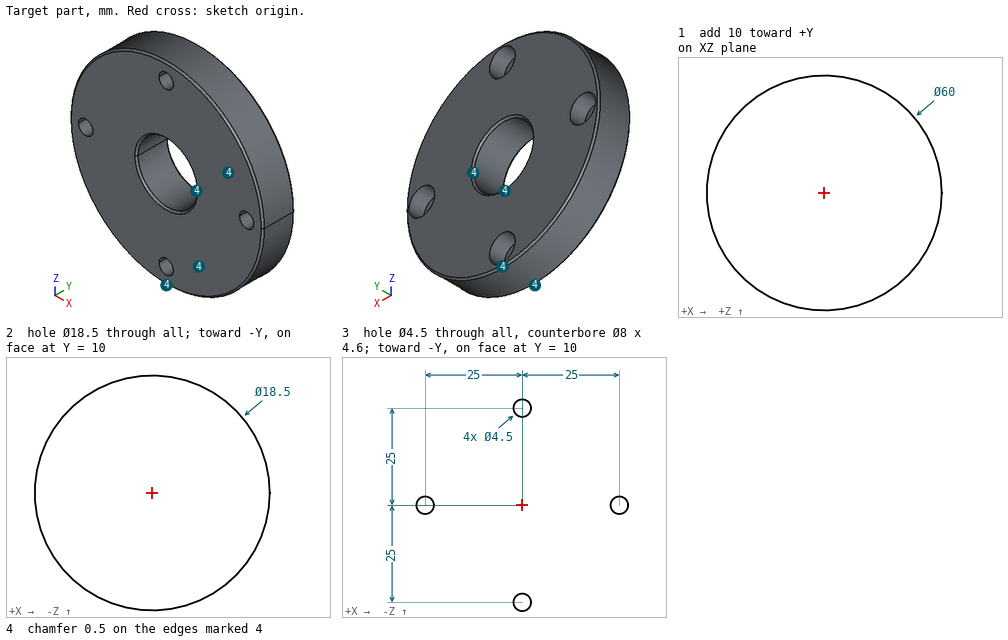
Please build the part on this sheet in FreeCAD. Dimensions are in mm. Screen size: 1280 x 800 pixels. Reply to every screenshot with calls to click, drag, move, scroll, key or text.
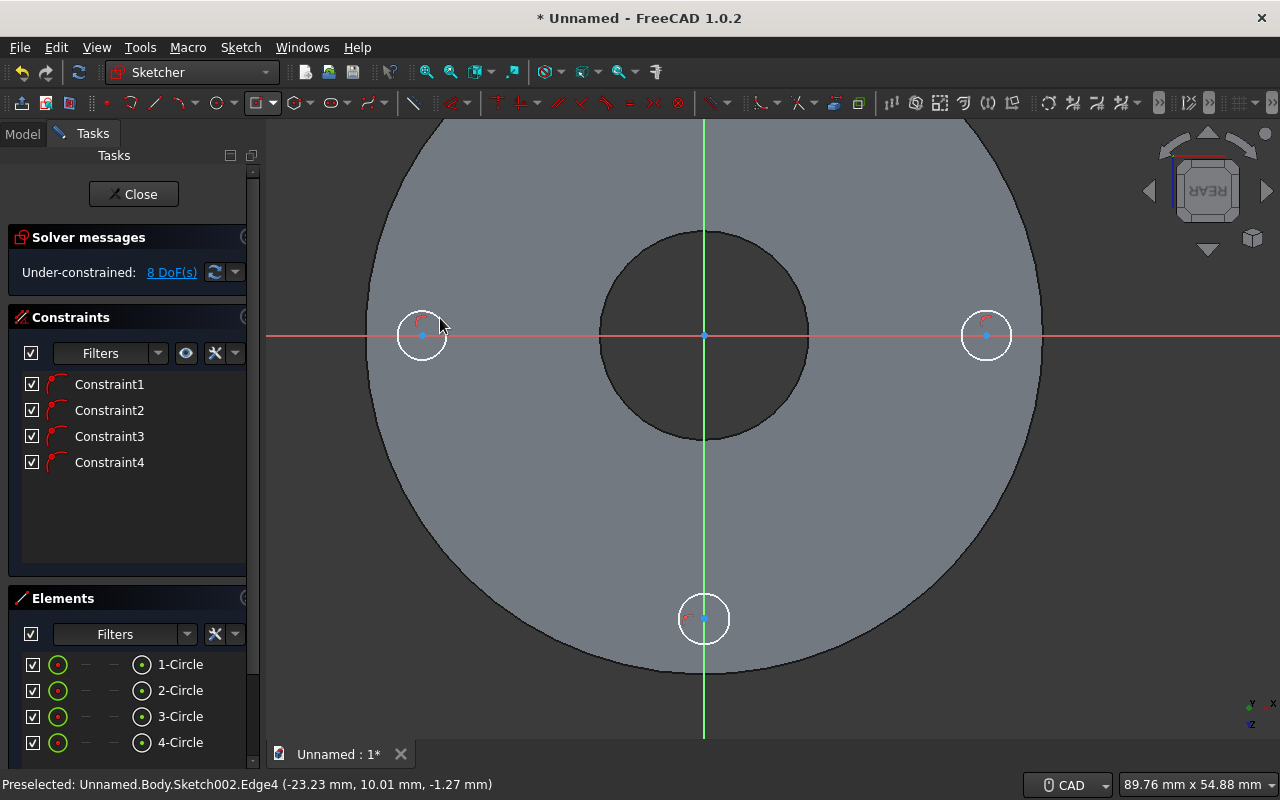
scroll(705, 619, down, 2)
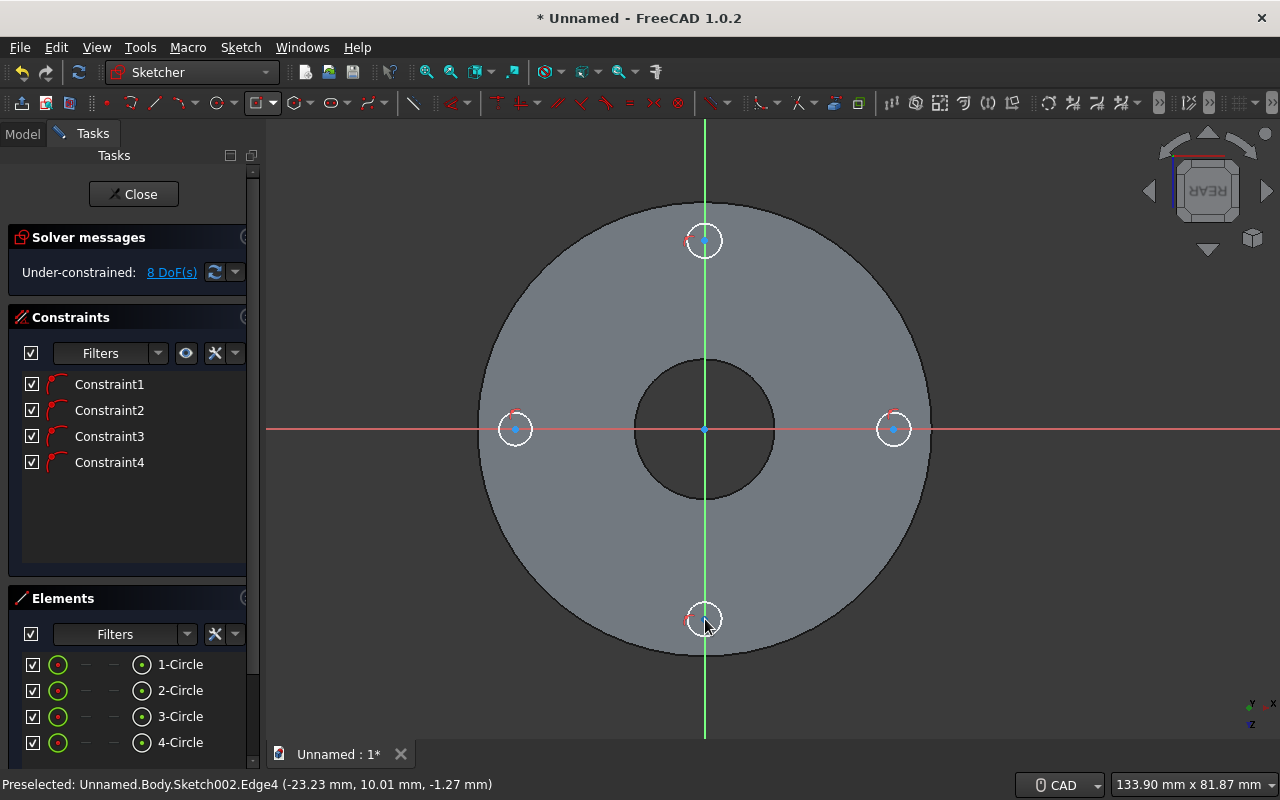
click(717, 228)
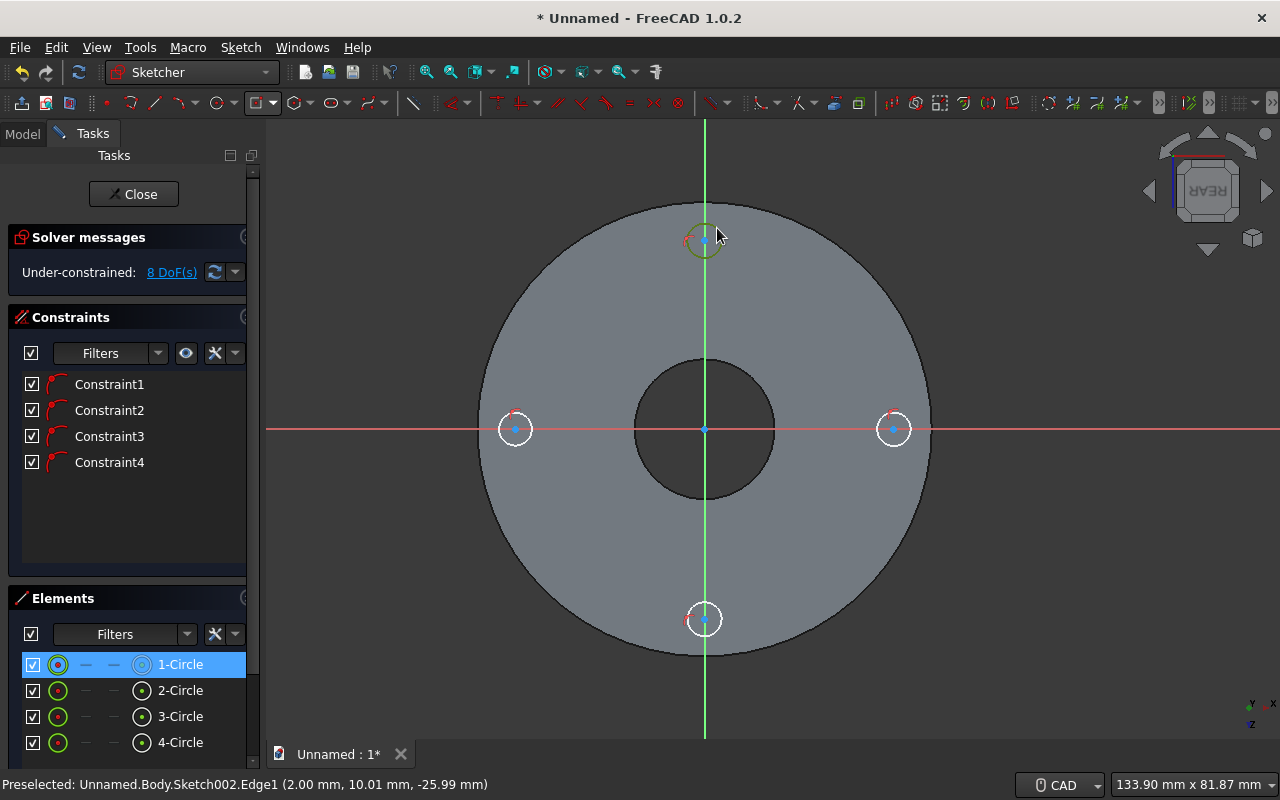
click(906, 417)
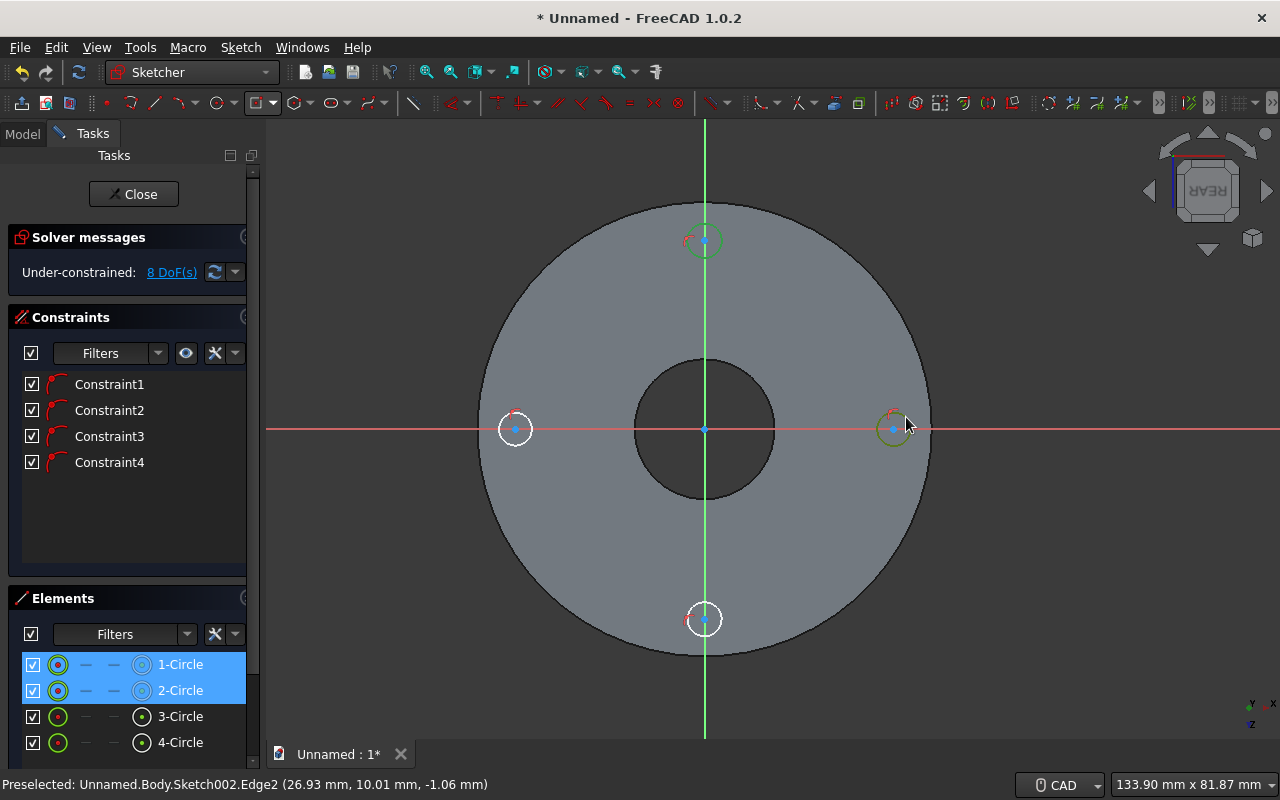
click(717, 607)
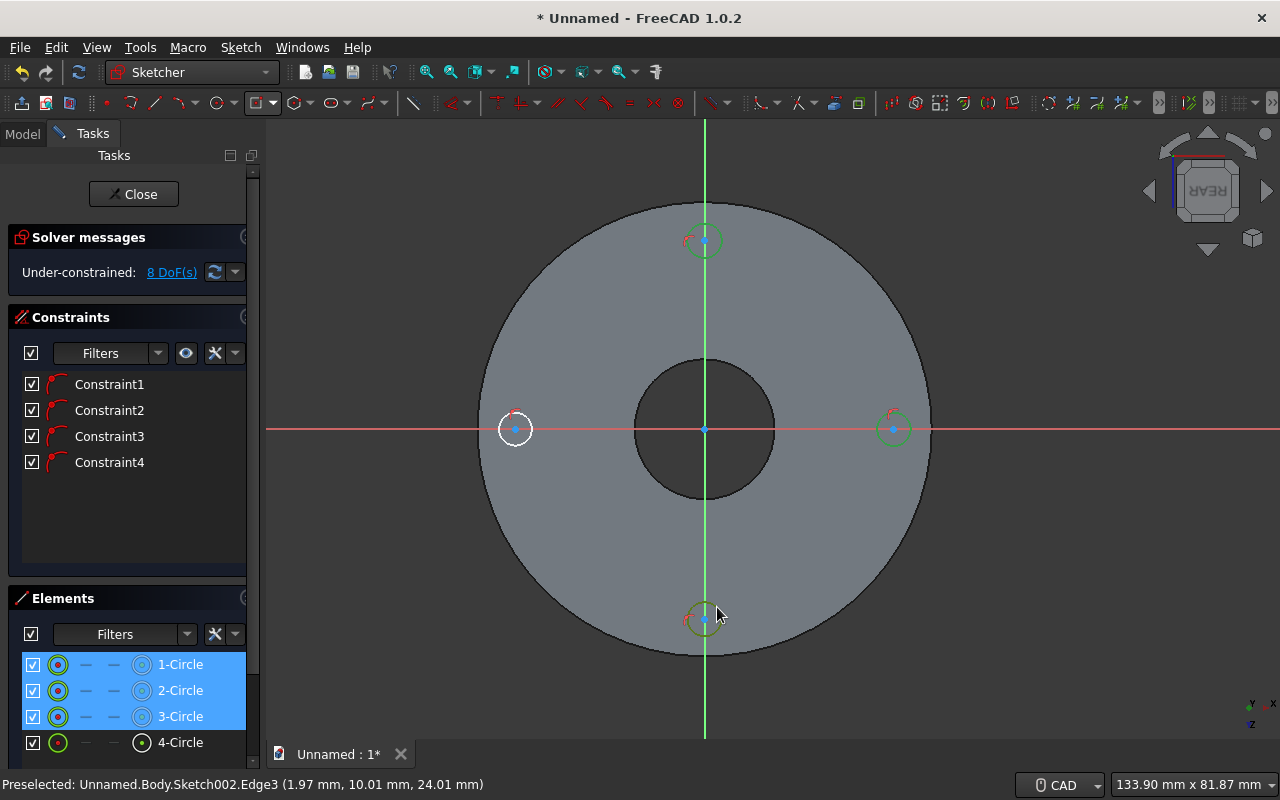
click(527, 418)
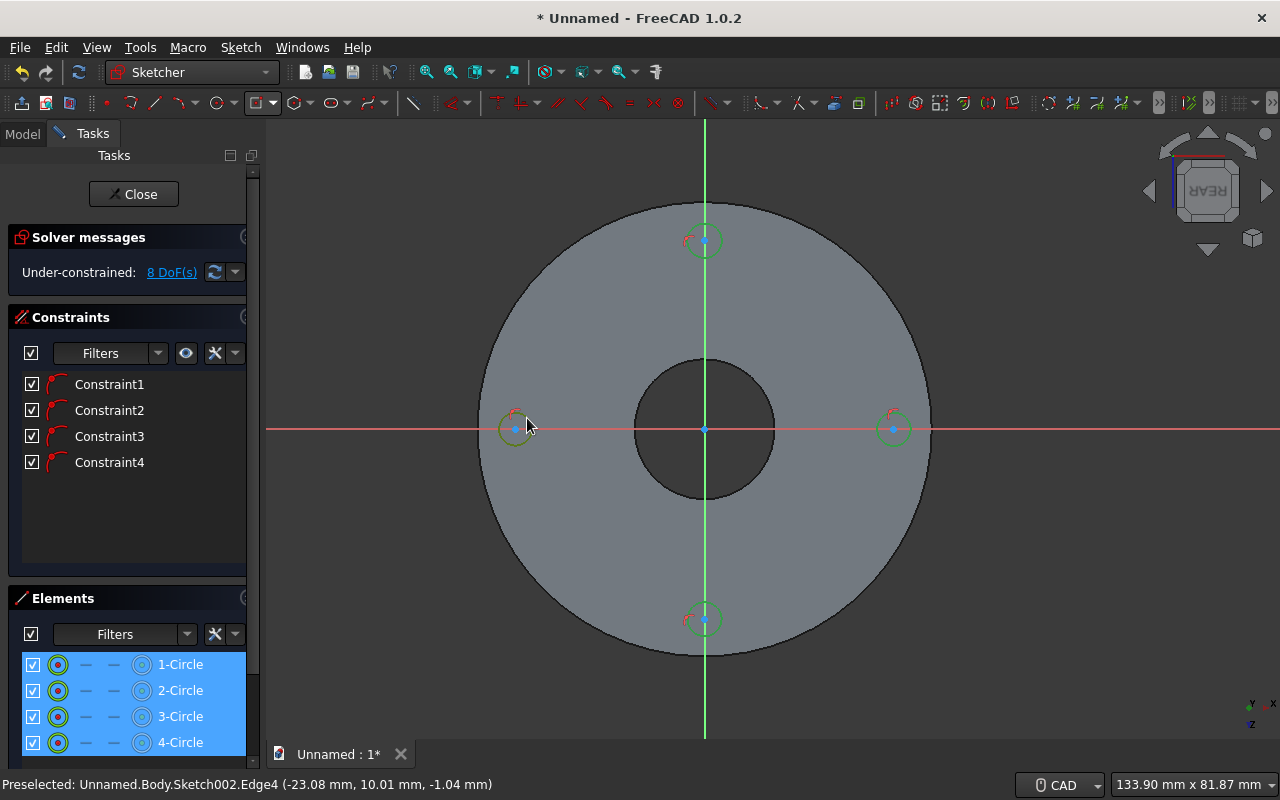
key(e)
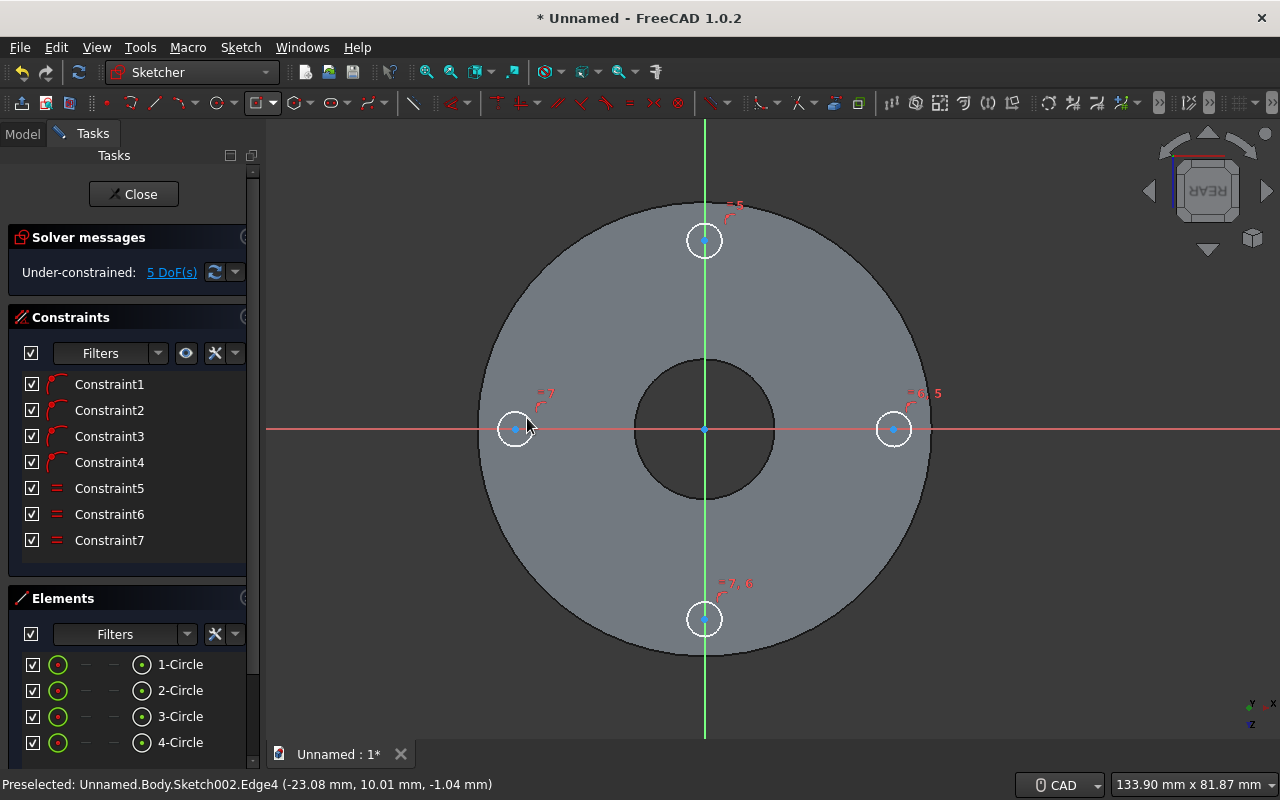
key(d)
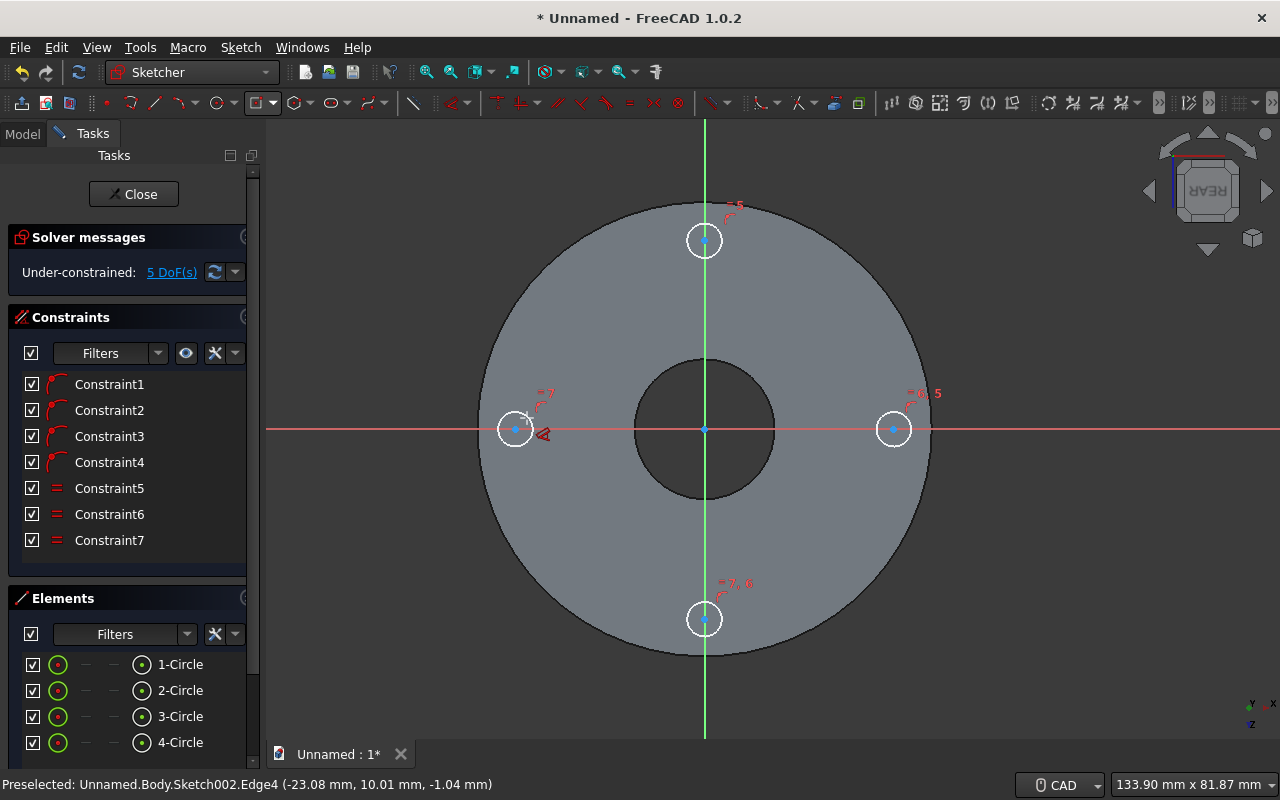
click(717, 228)
click(739, 205)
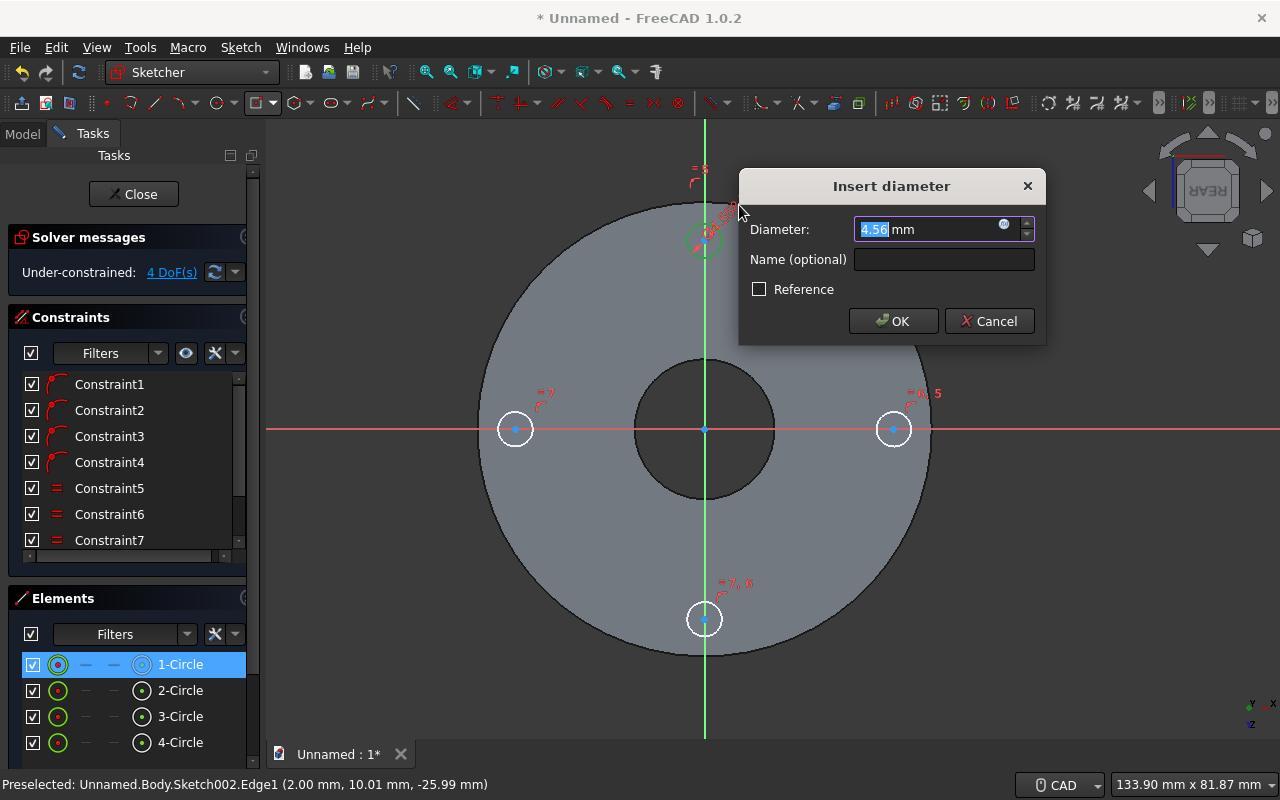
text(4.5)
key(Return)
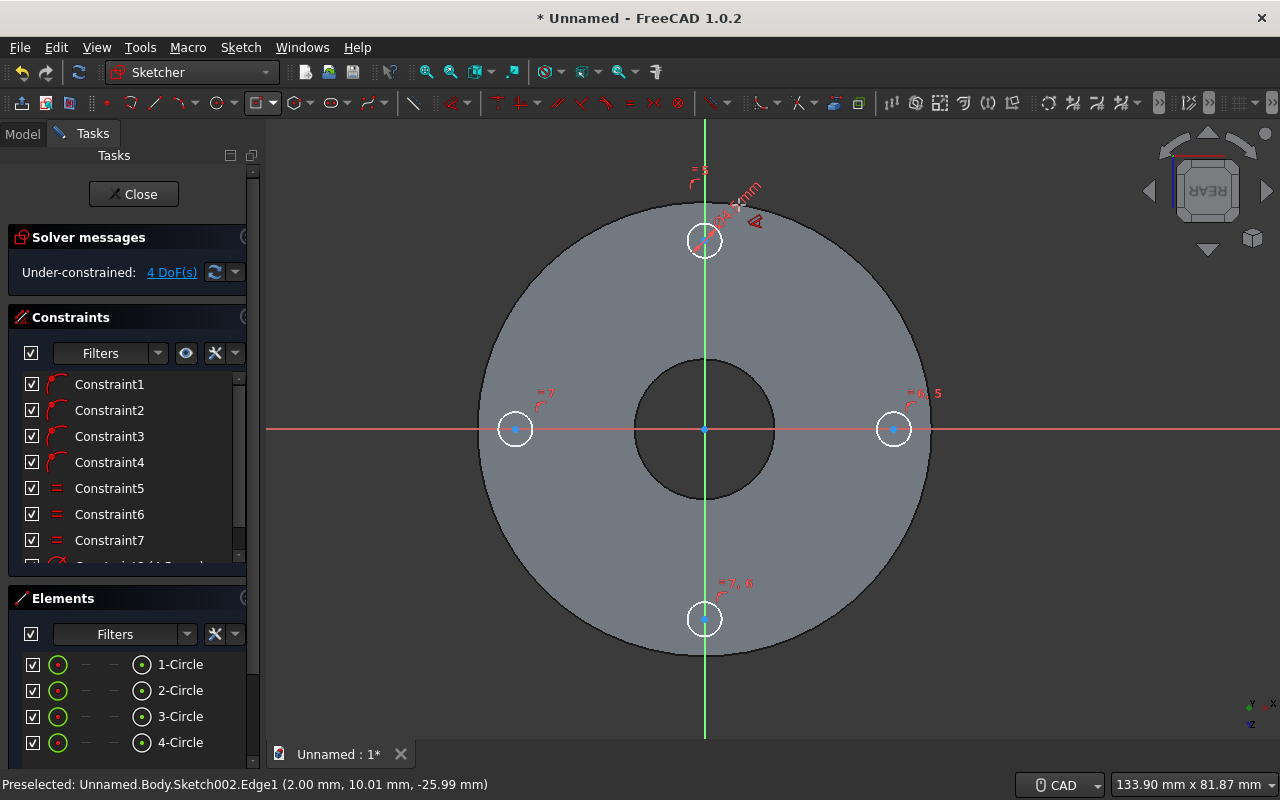
click(705, 241)
click(739, 335)